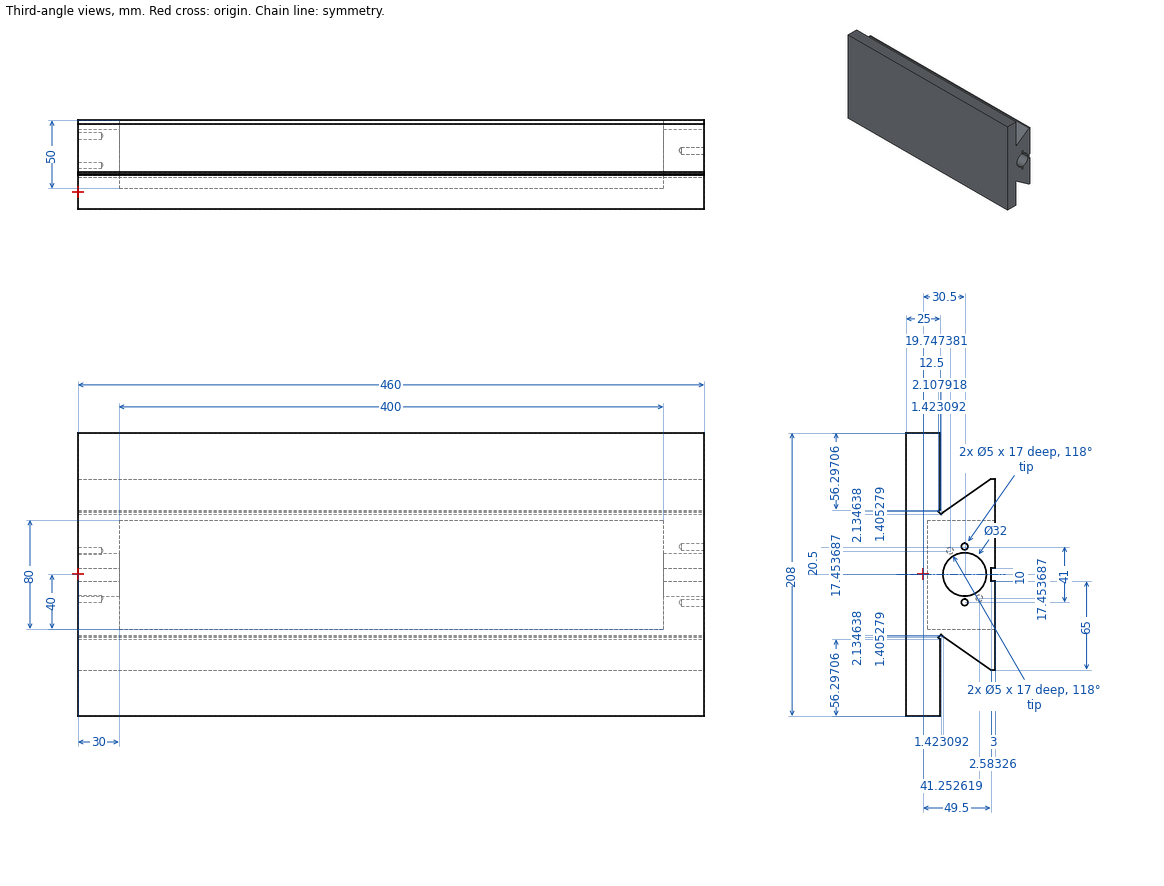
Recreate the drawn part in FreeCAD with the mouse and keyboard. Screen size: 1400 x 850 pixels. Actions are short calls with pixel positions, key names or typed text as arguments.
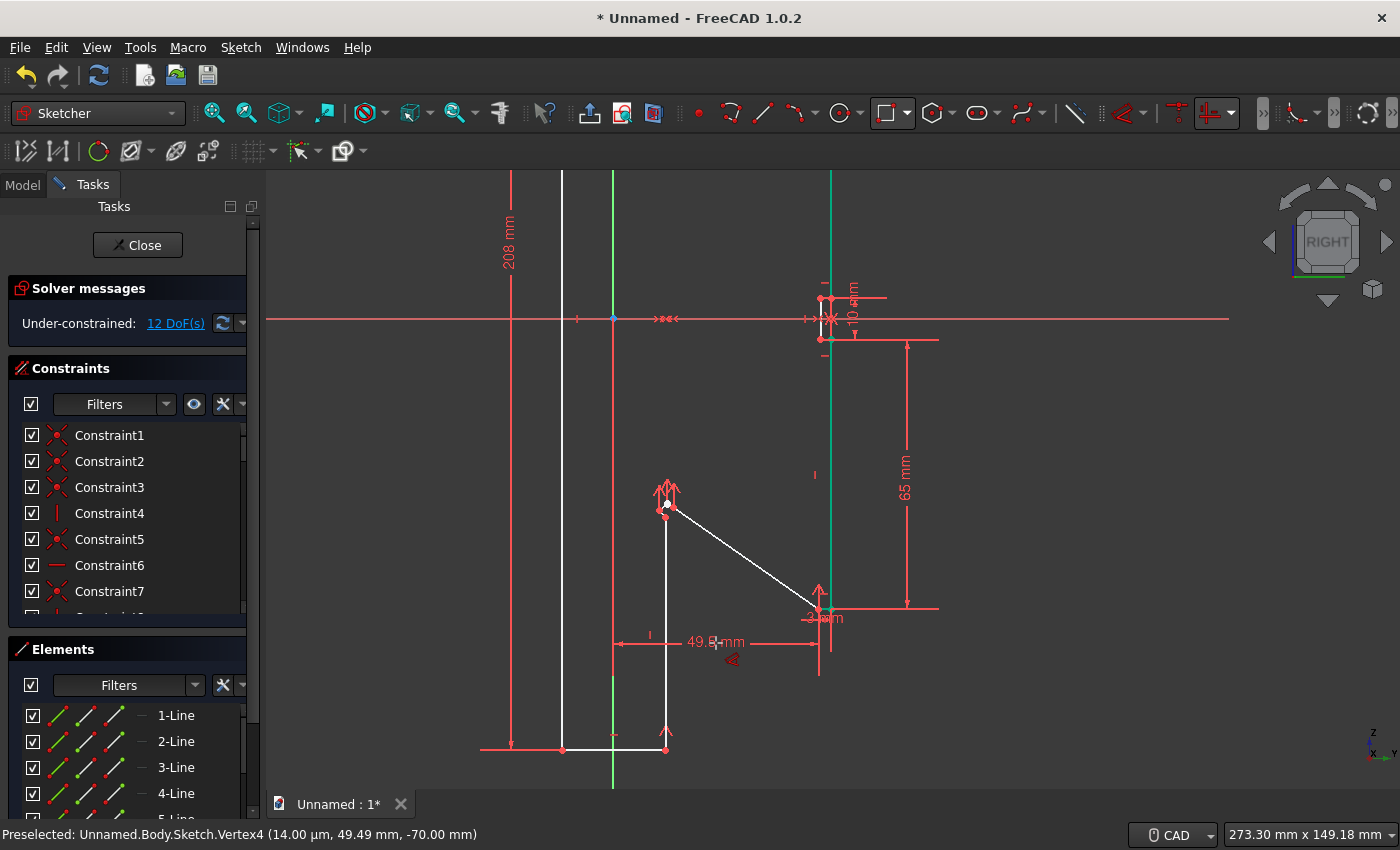
scroll(820, 611, down, 4)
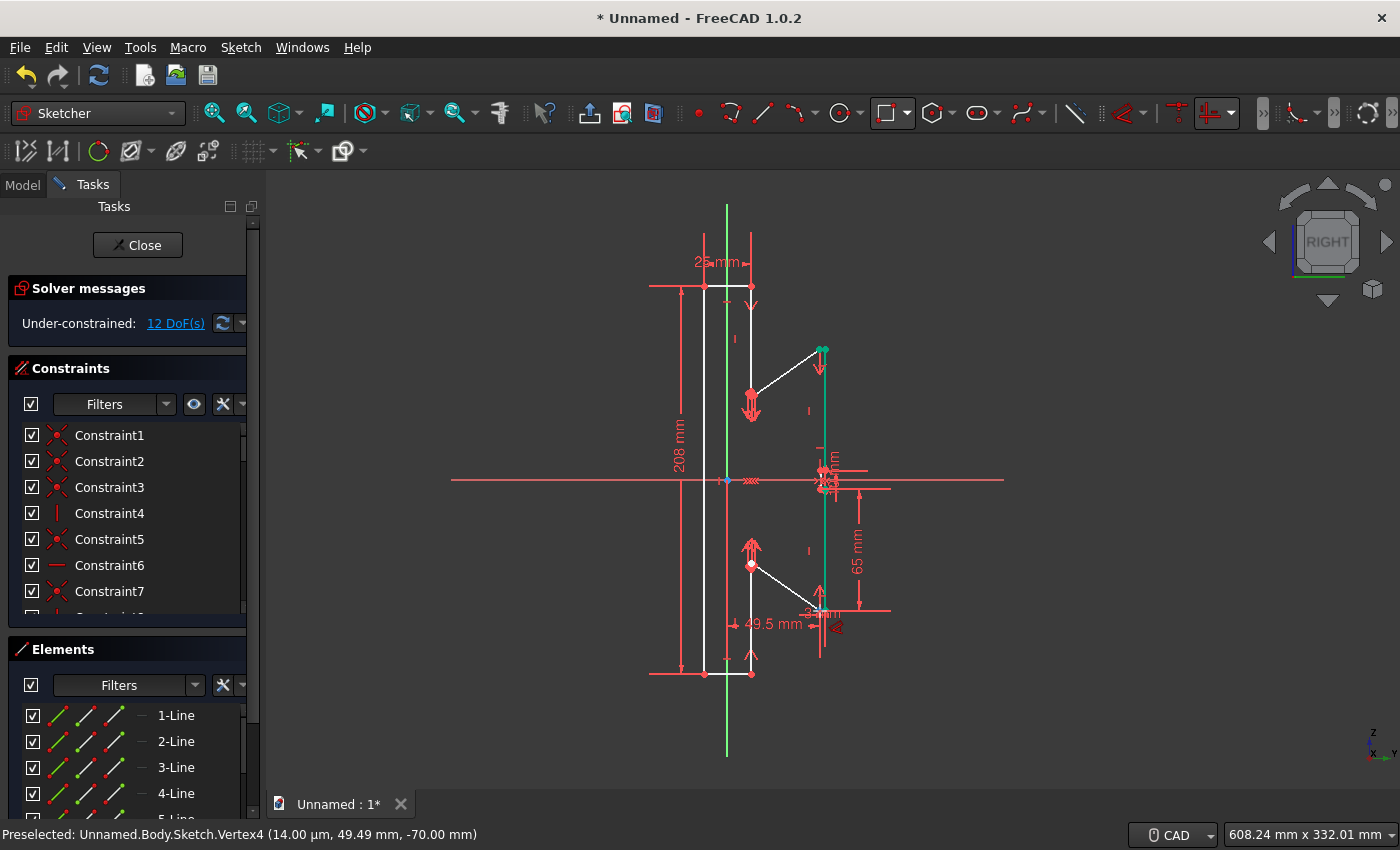
scroll(751, 391, up, 6)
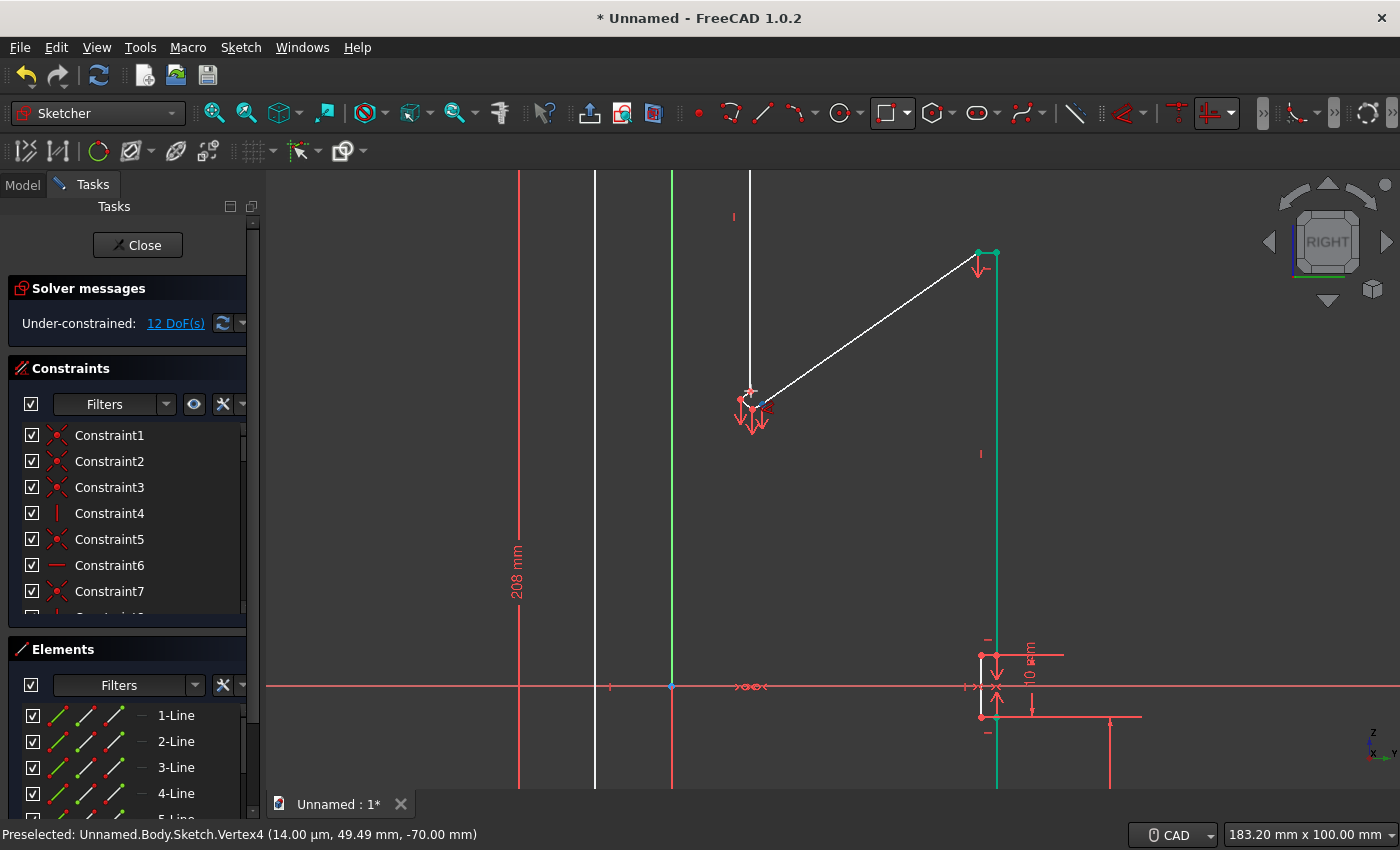
click(750, 391)
click(711, 357)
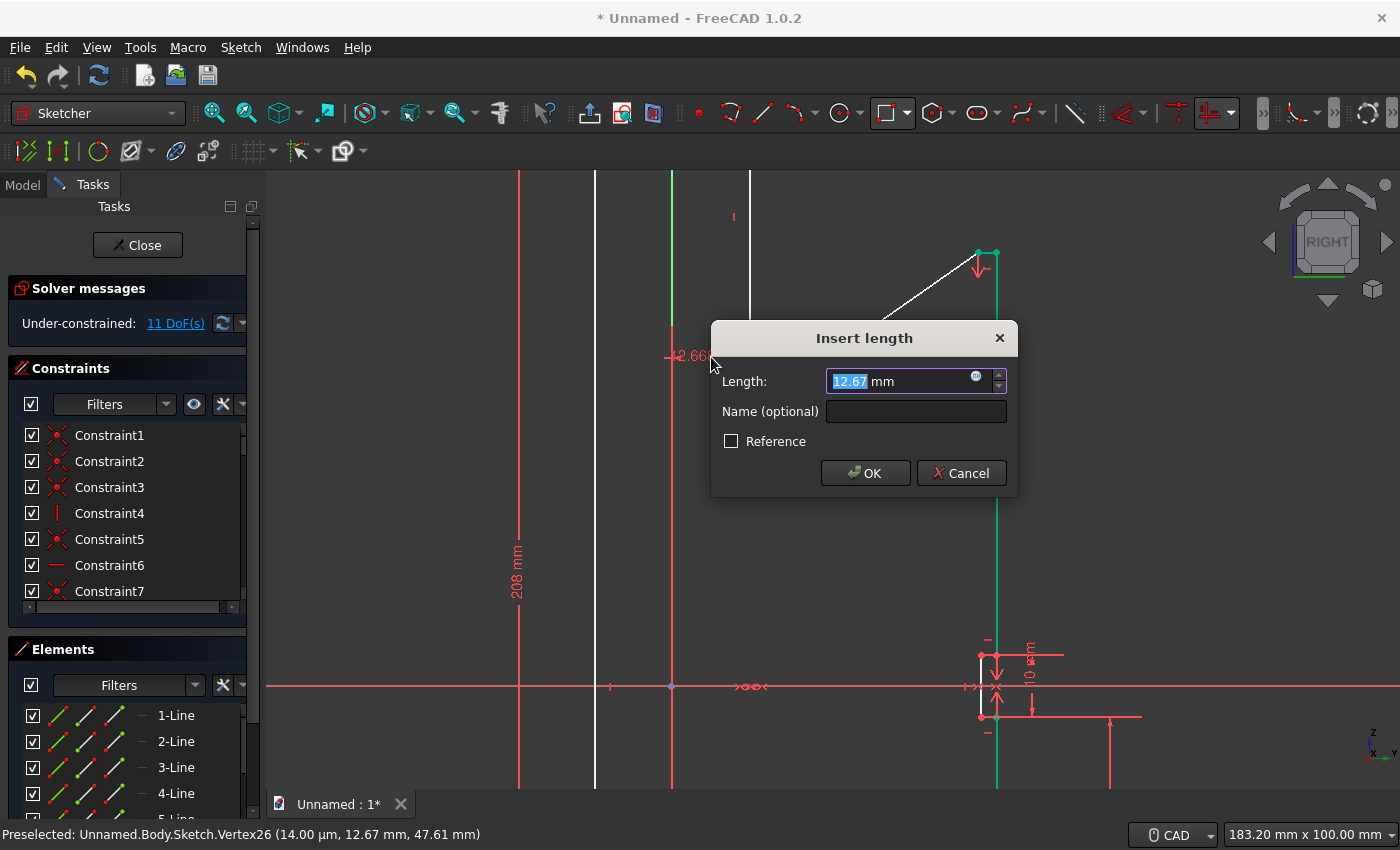
text(12.5)
key(Return)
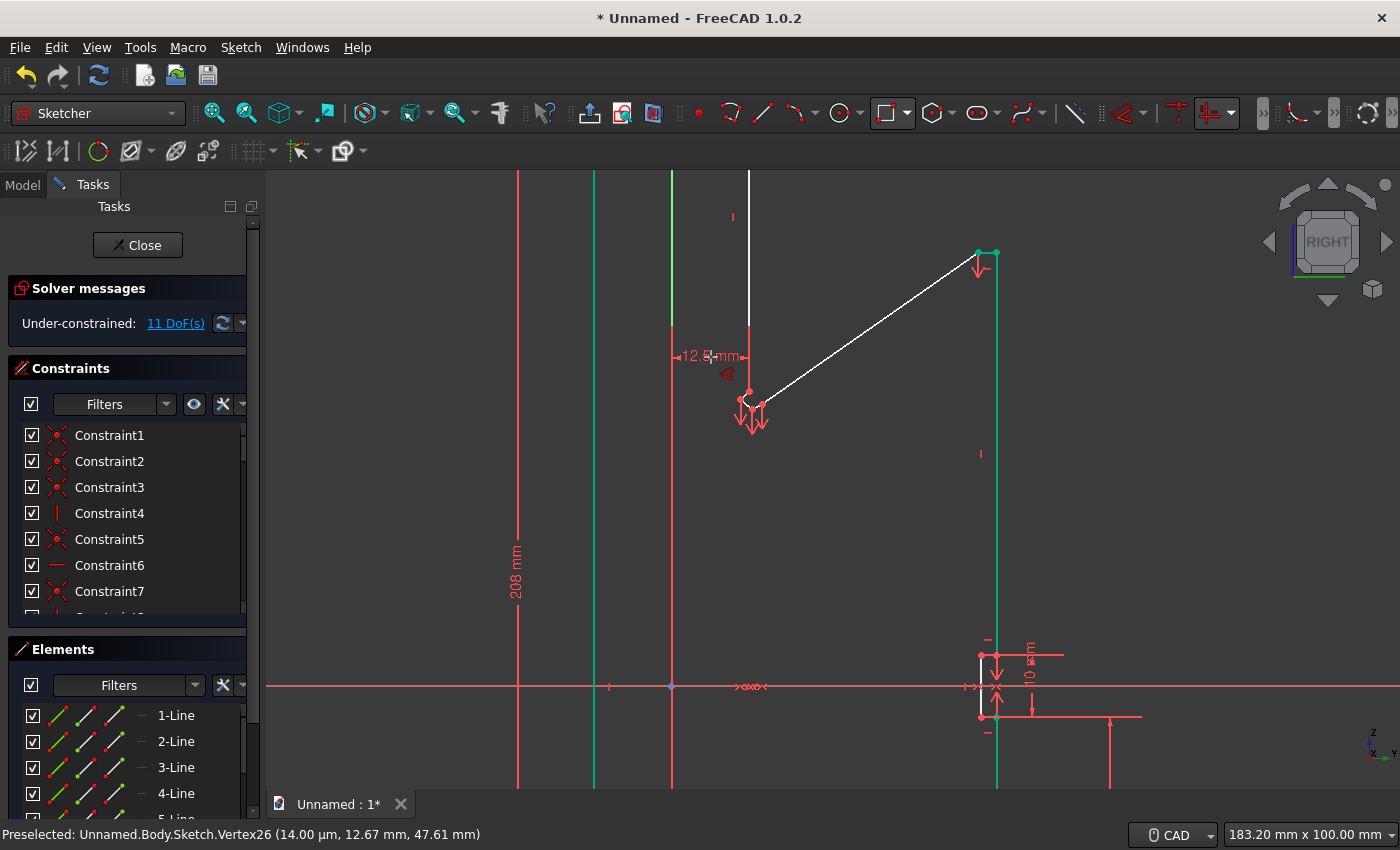
scroll(989, 717, up, 5)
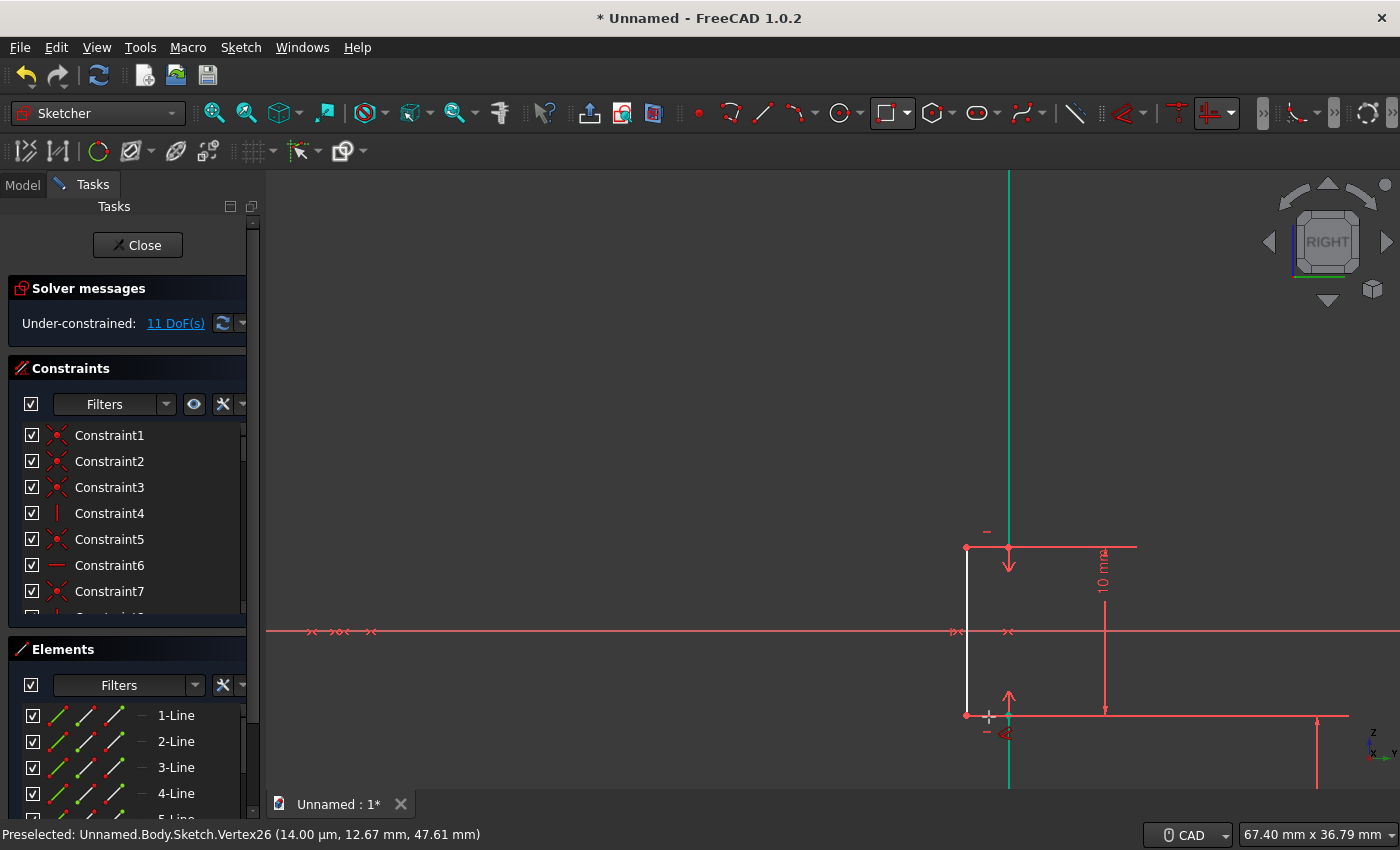
click(988, 716)
click(988, 750)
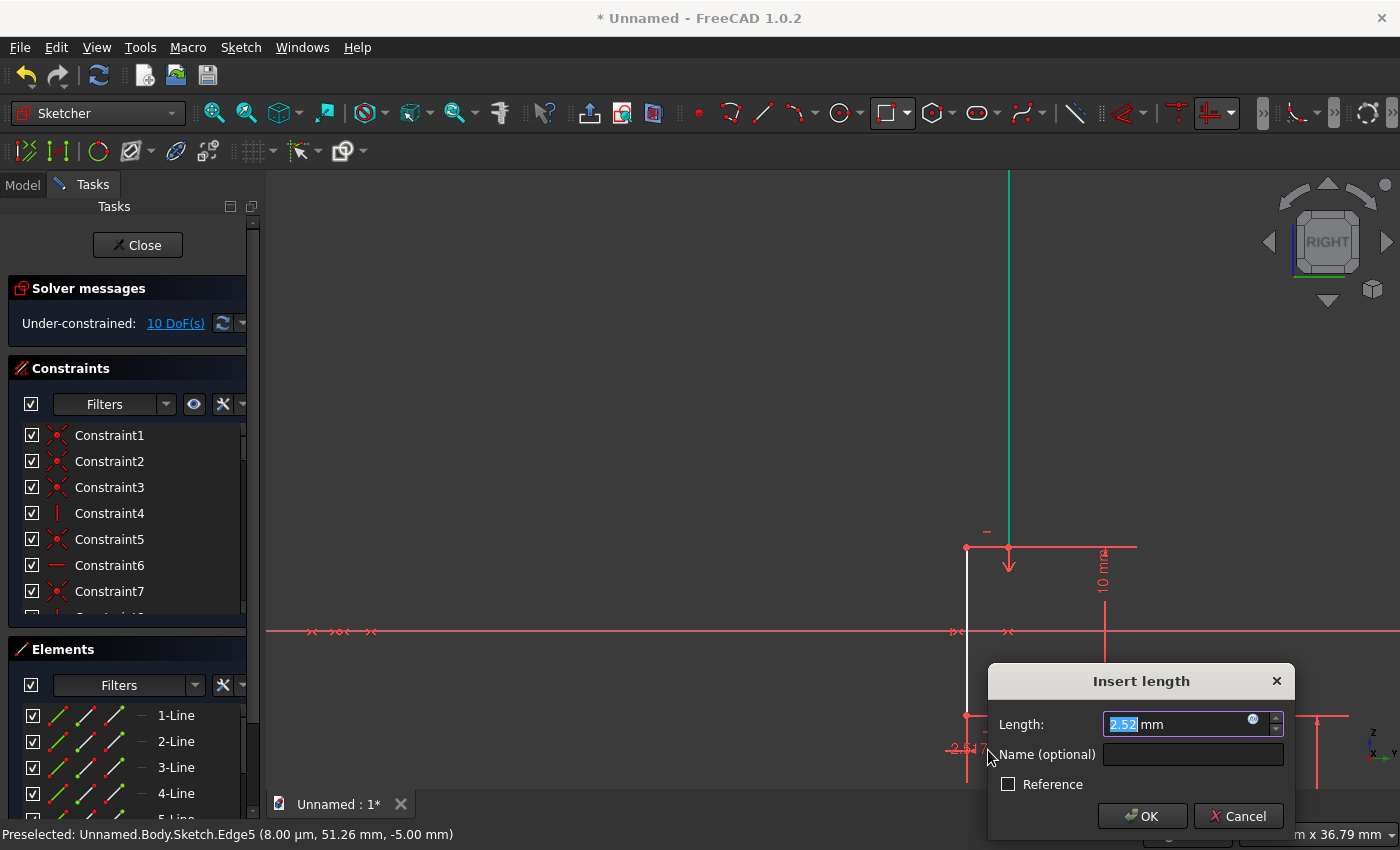
text(2.58326)
key(Return)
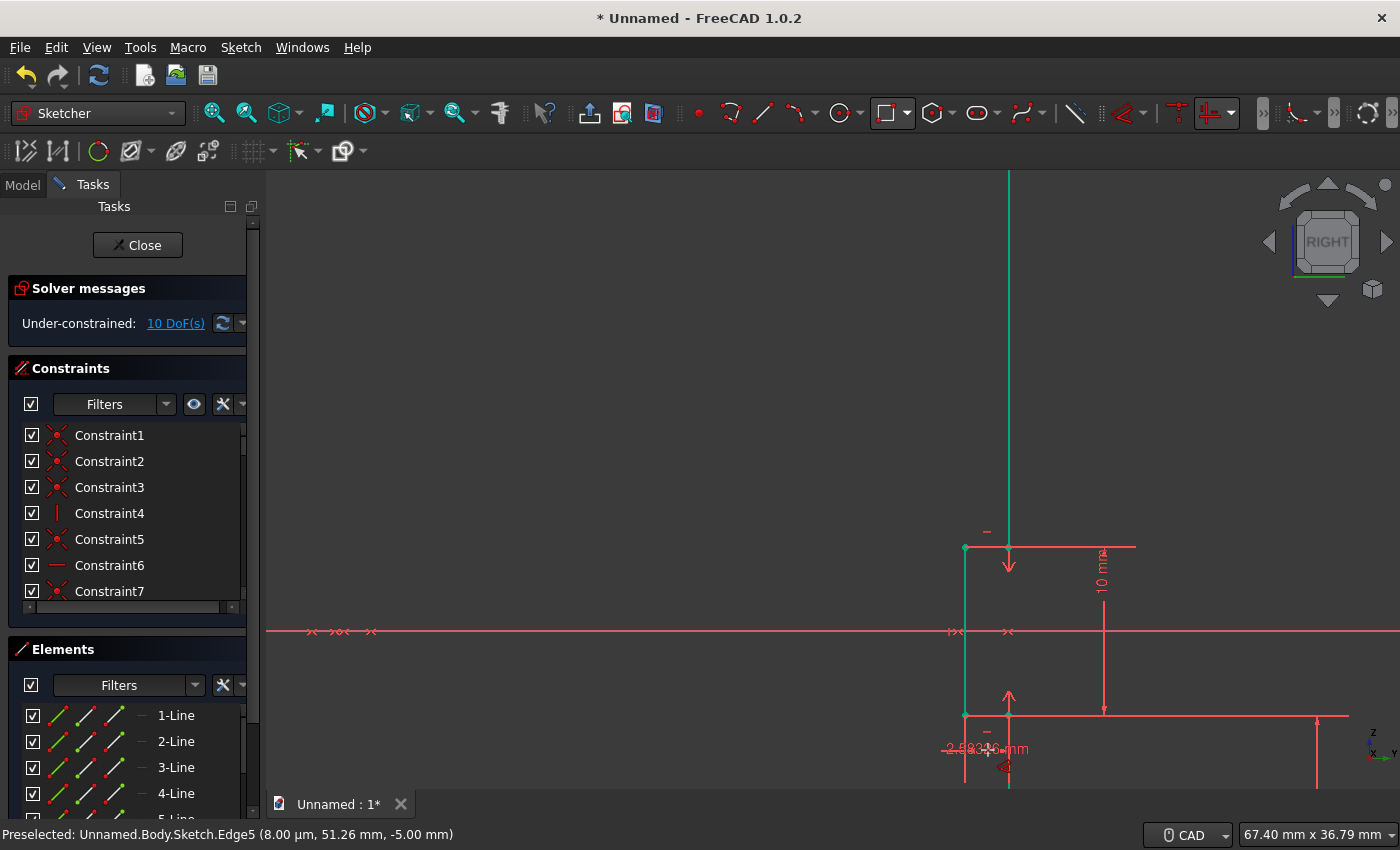
scroll(802, 461, down, 11)